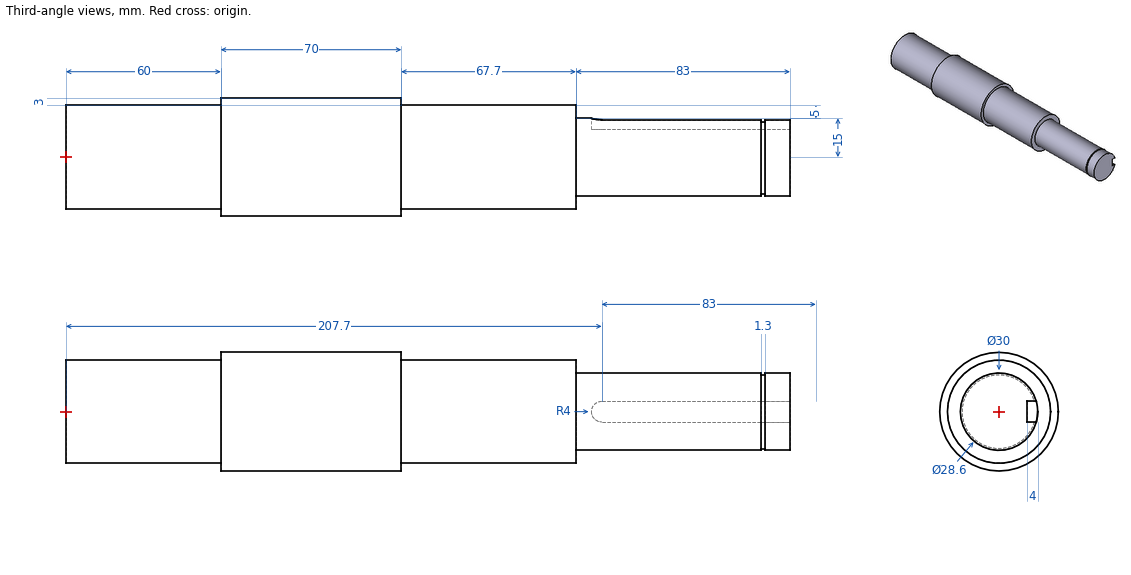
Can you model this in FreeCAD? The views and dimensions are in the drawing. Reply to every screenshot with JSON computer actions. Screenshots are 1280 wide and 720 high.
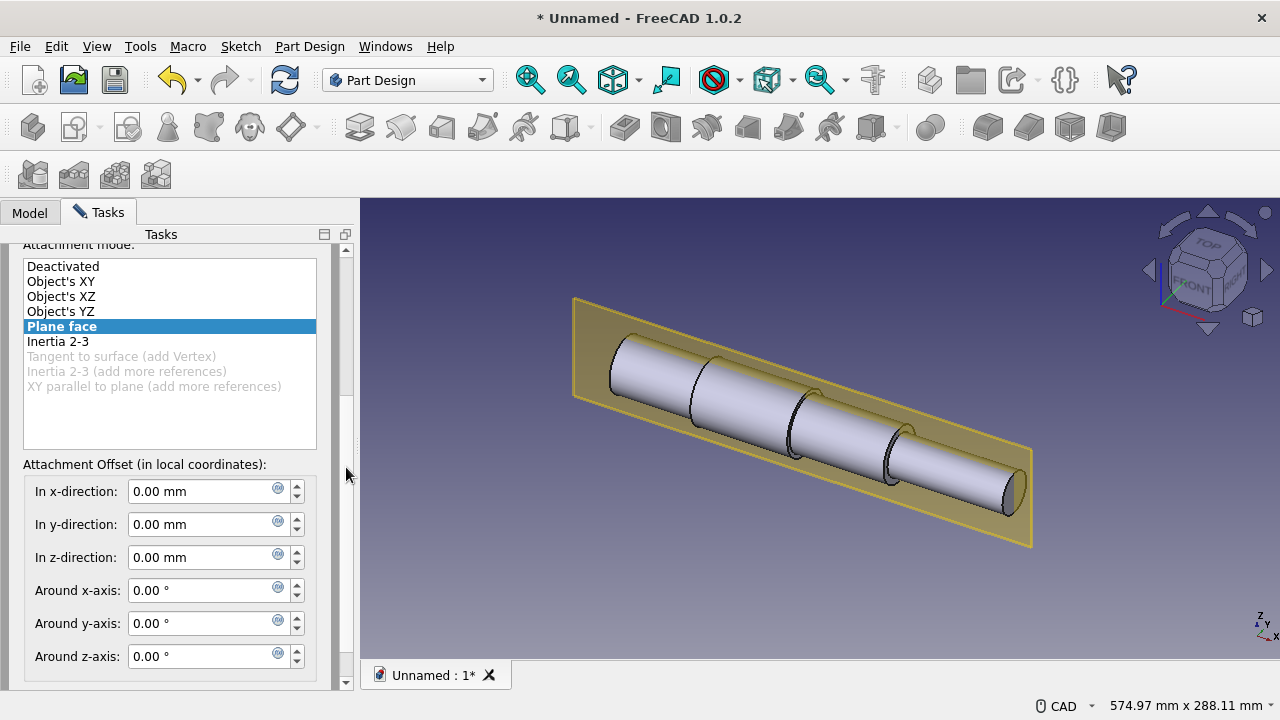
{"action": "triple_click", "coordinate": [210, 558]}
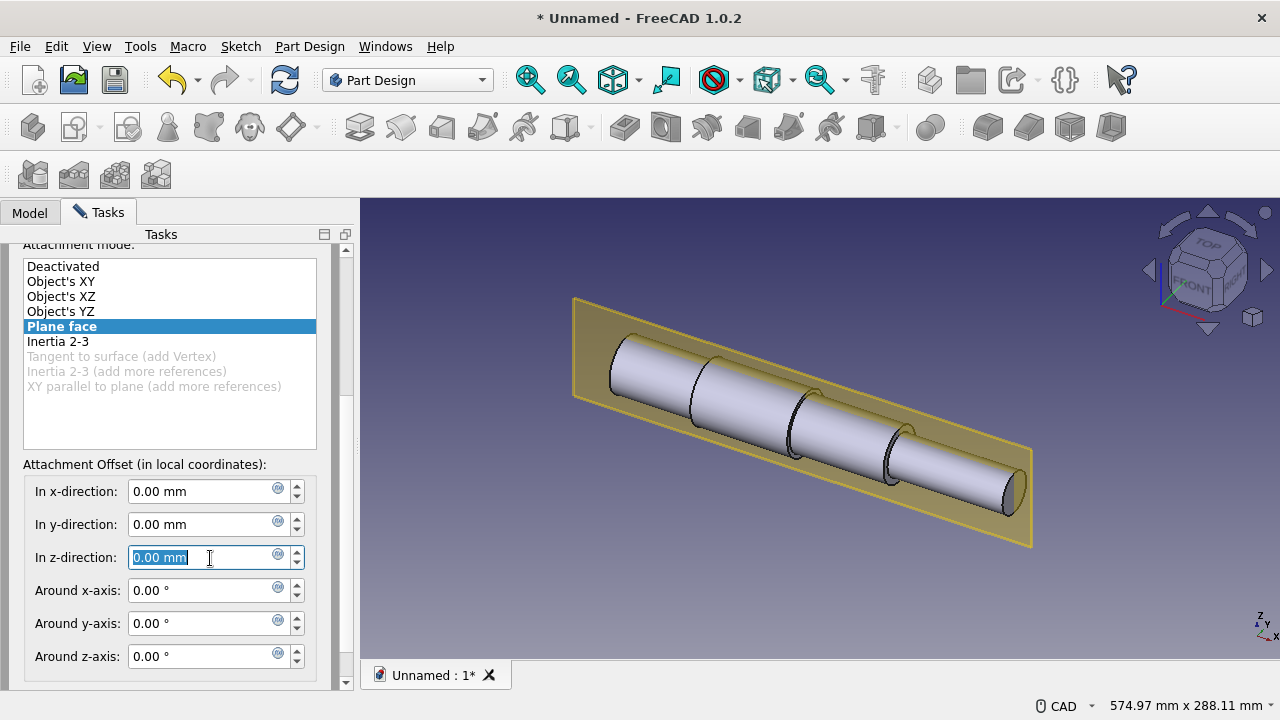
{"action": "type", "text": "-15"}
{"action": "key", "text": "Tab"}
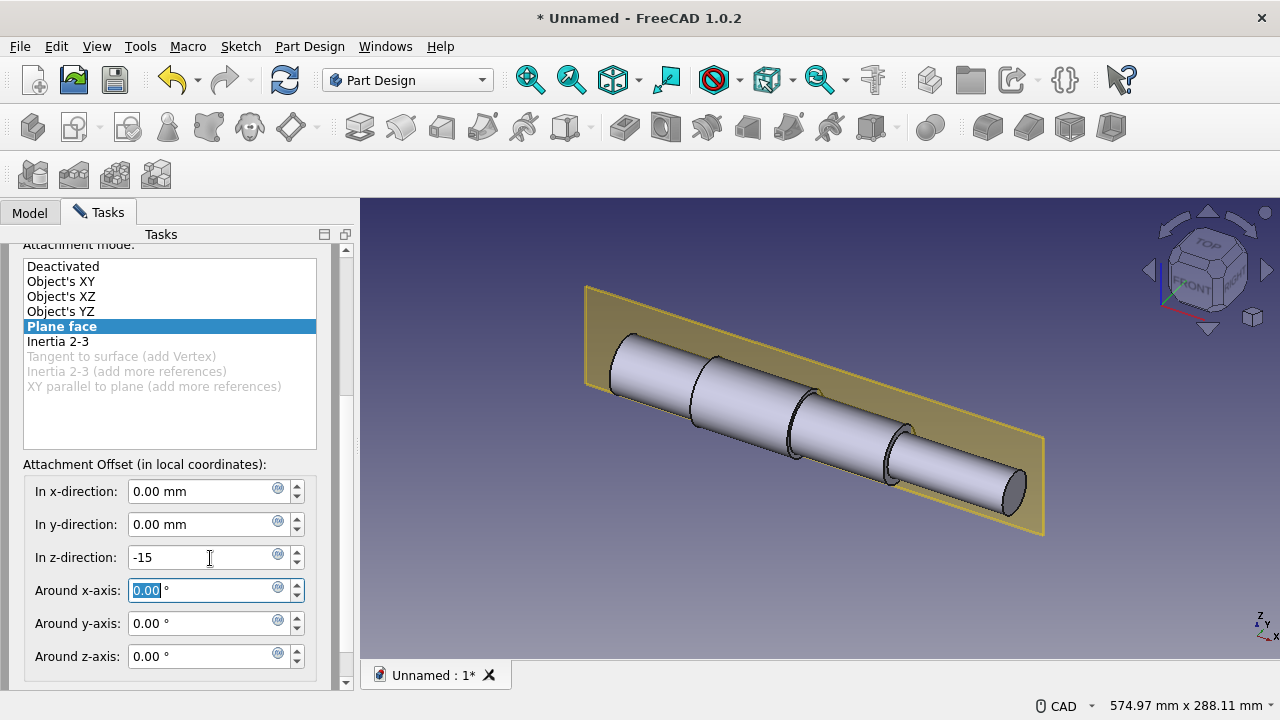
{"action": "scroll", "coordinate": [346, 467], "scroll_direction": "up", "scroll_amount": 5}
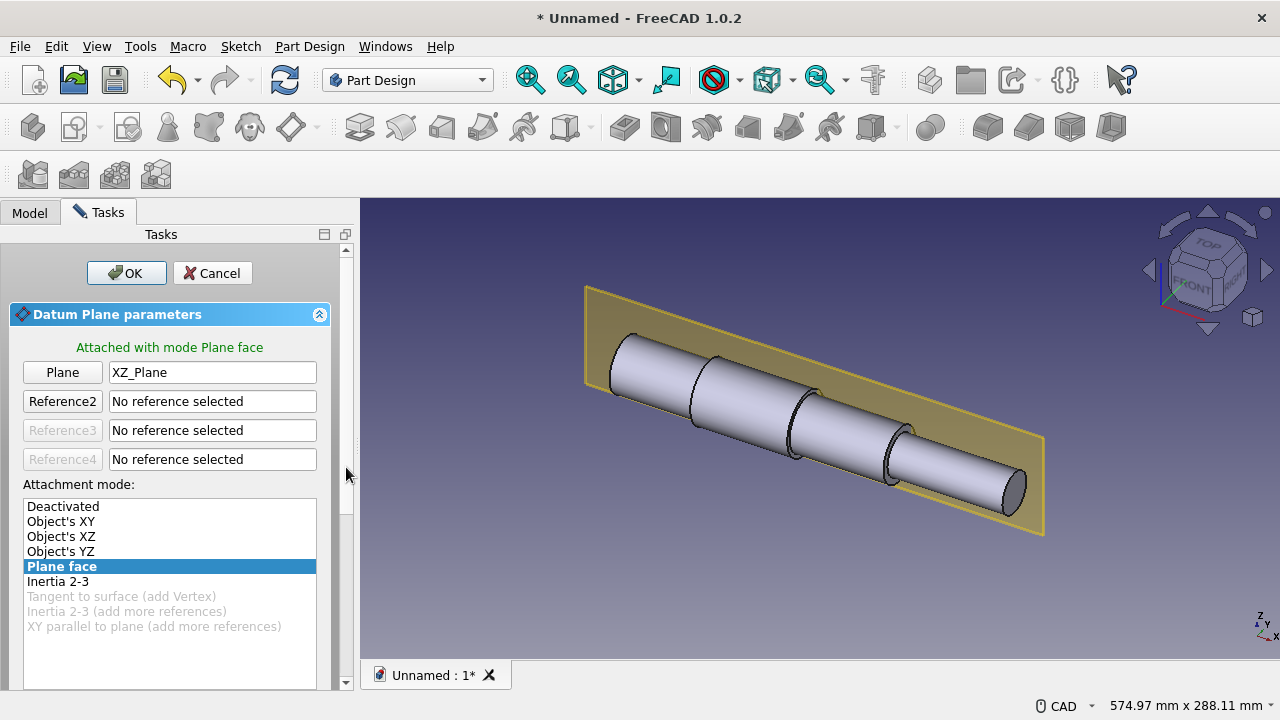
{"action": "left_click", "coordinate": [127, 273]}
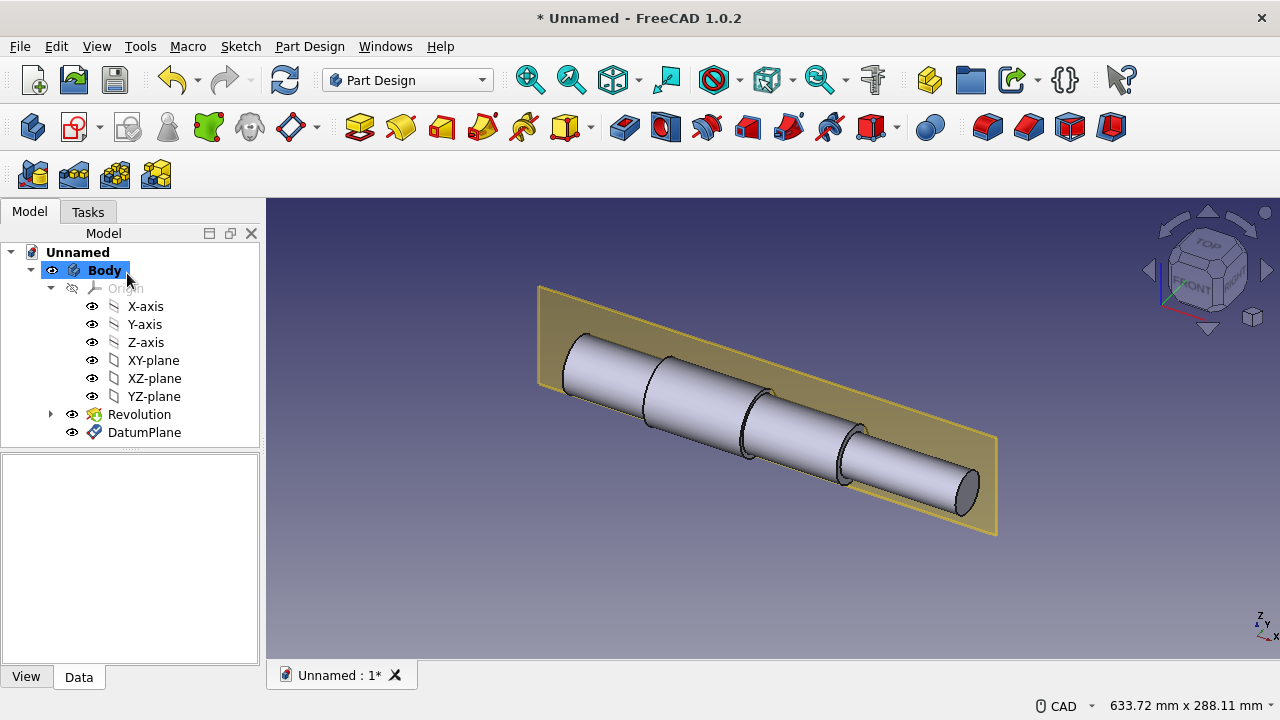
{"action": "left_click", "coordinate": [117, 432]}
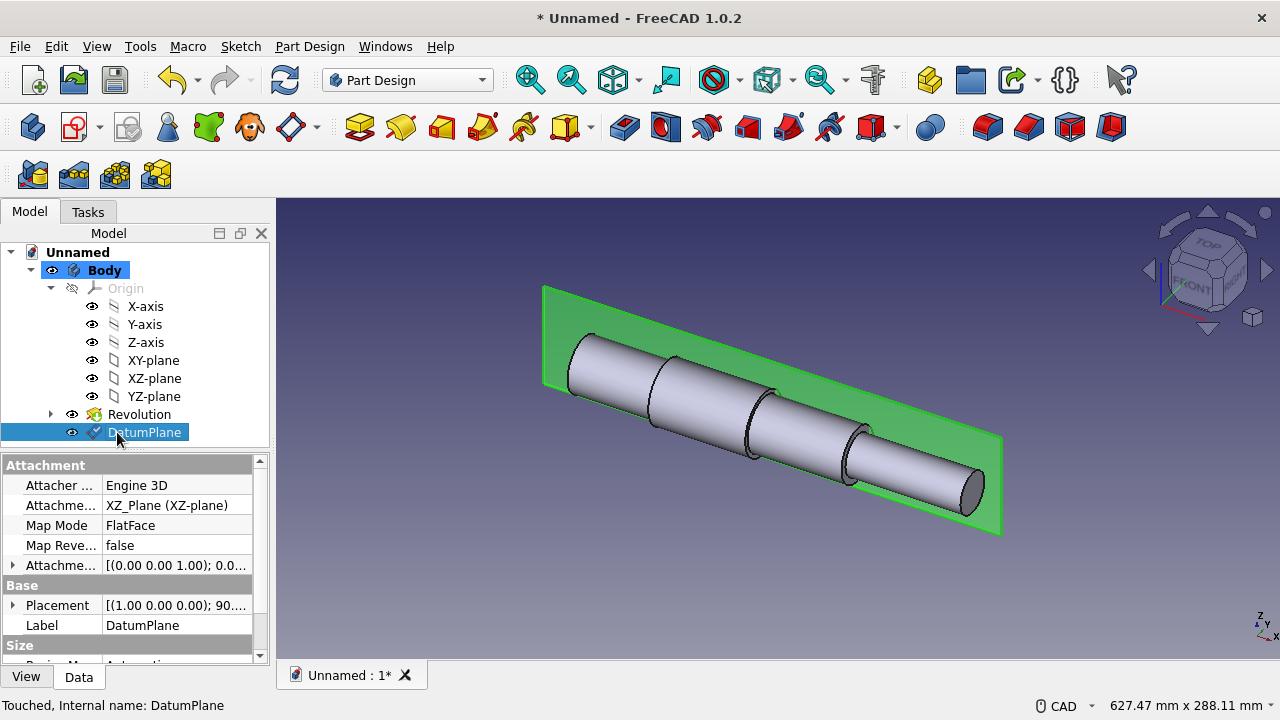
{"action": "left_click", "coordinate": [74, 128]}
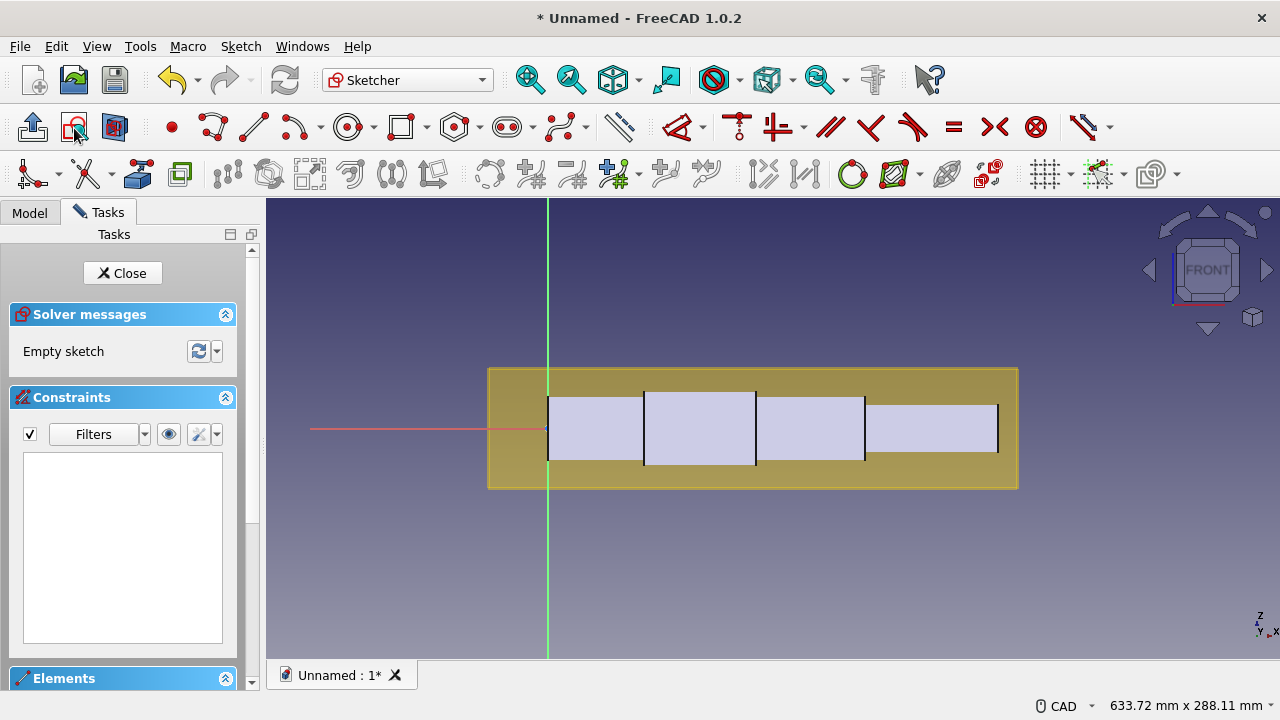
{"action": "key", "text": "q s"}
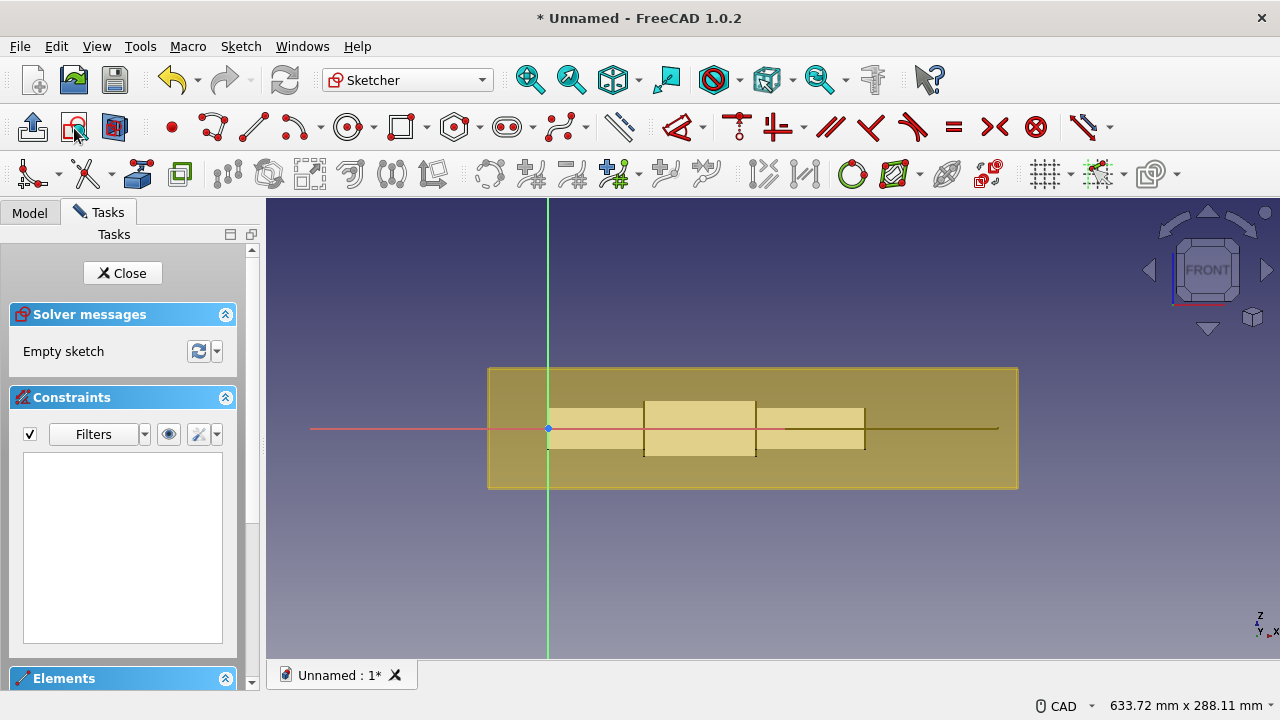
{"action": "scroll", "coordinate": [1022, 429], "scroll_direction": "up", "scroll_amount": 7}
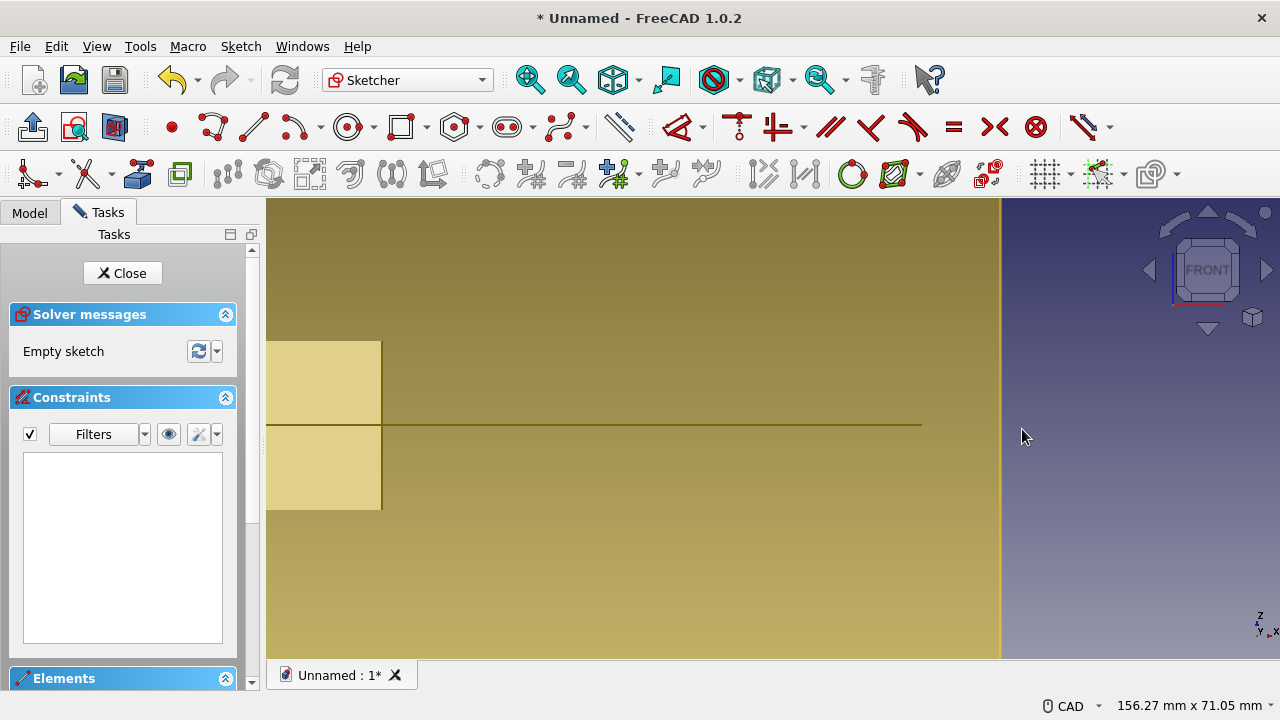
{"action": "key", "text": "g m"}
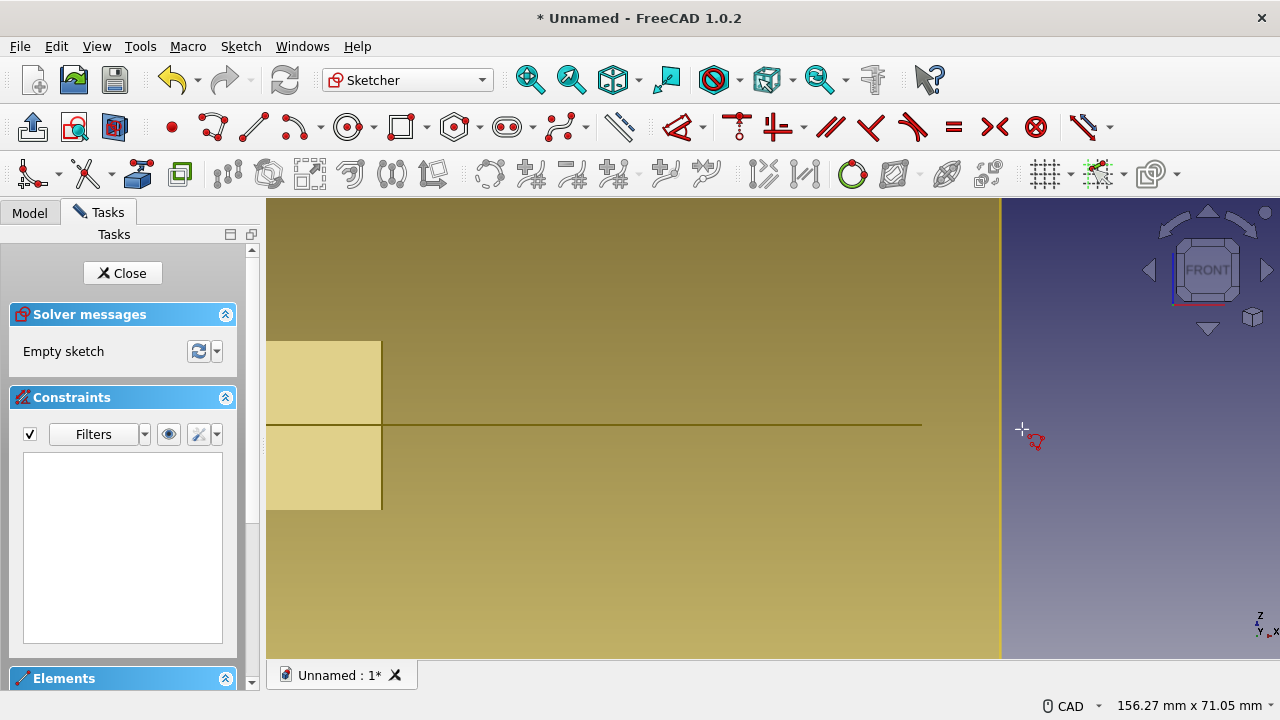
{"action": "left_click", "coordinate": [447, 399]}
{"action": "left_click", "coordinate": [986, 399]}
{"action": "left_click", "coordinate": [986, 451]}
{"action": "left_click", "coordinate": [447, 451]}
{"action": "right_click", "coordinate": [447, 451]}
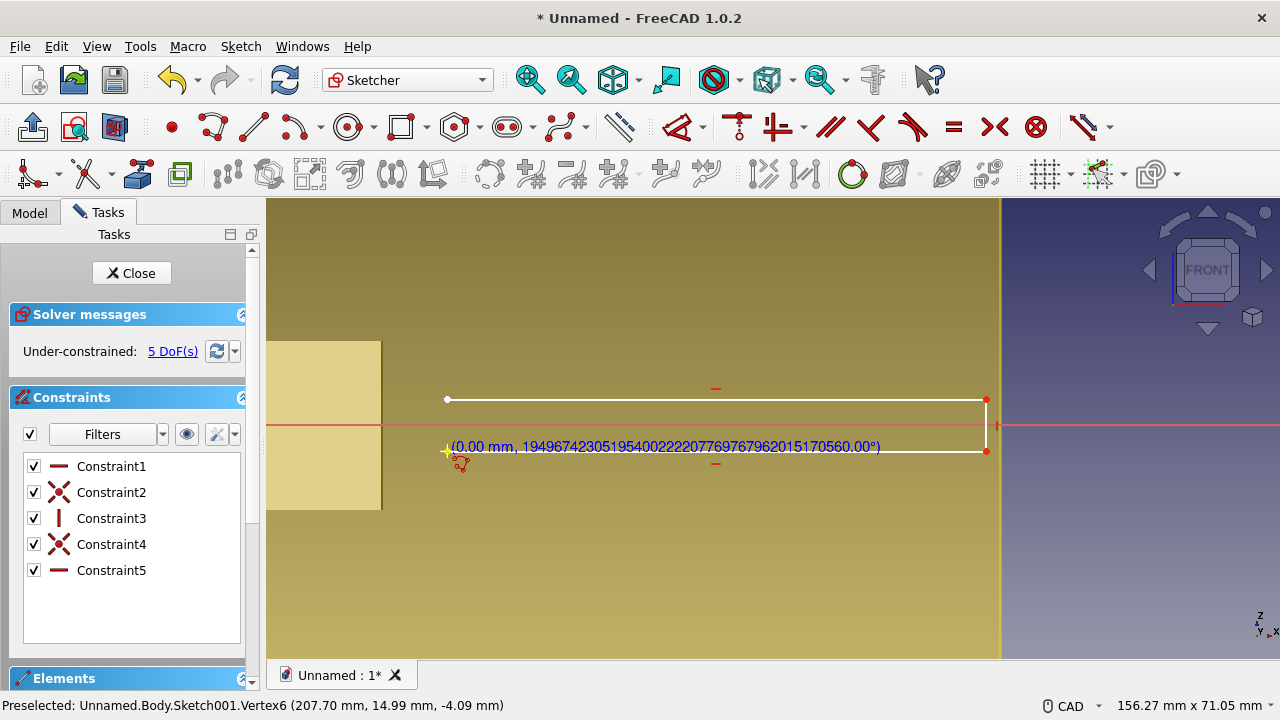
{"action": "key", "text": "g 3 a"}